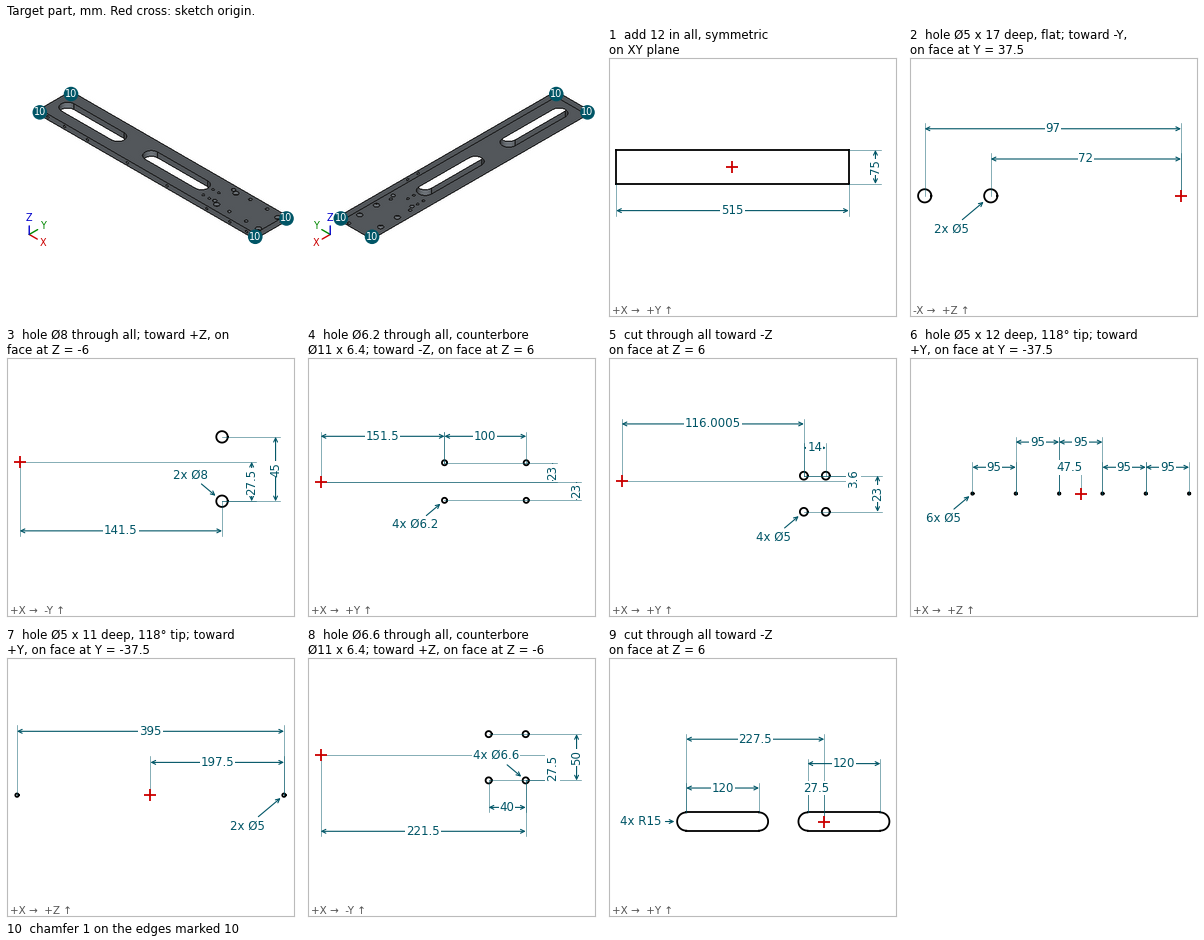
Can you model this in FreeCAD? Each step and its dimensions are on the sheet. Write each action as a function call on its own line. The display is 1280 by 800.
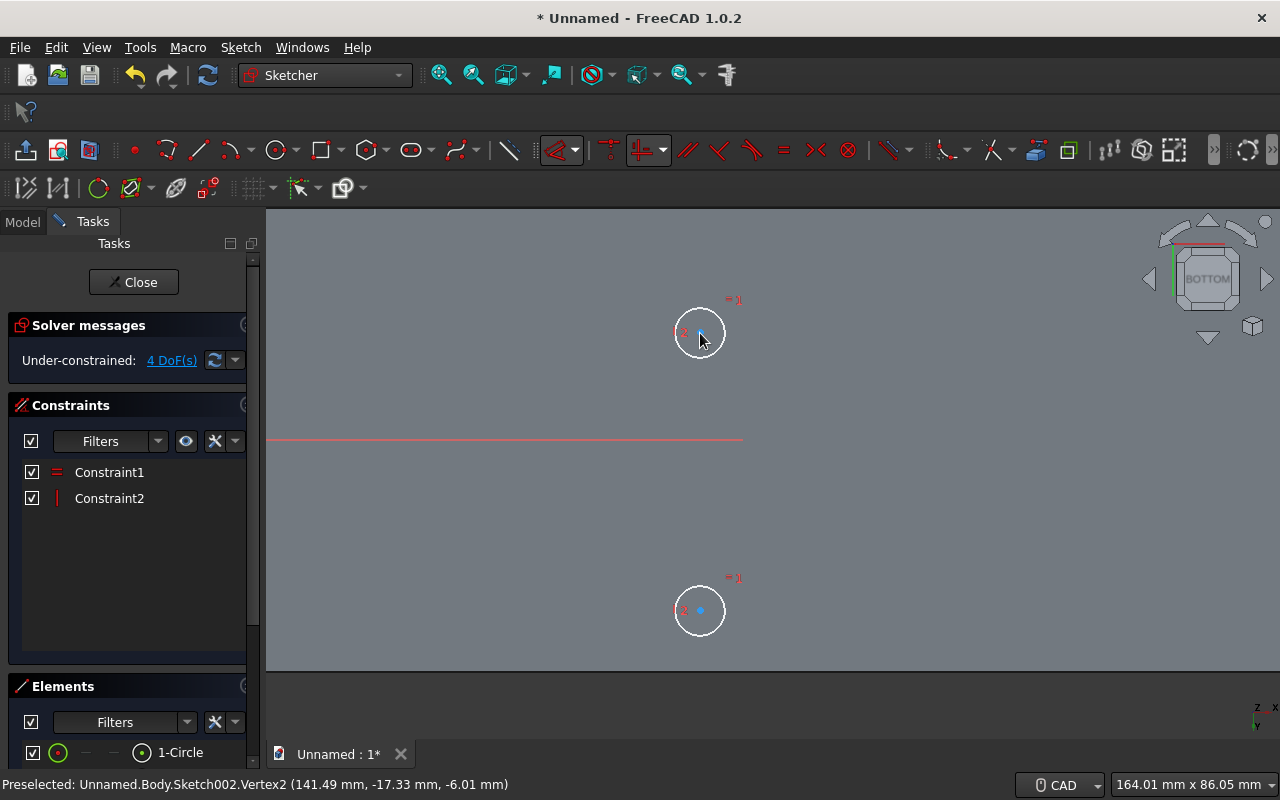
key(d)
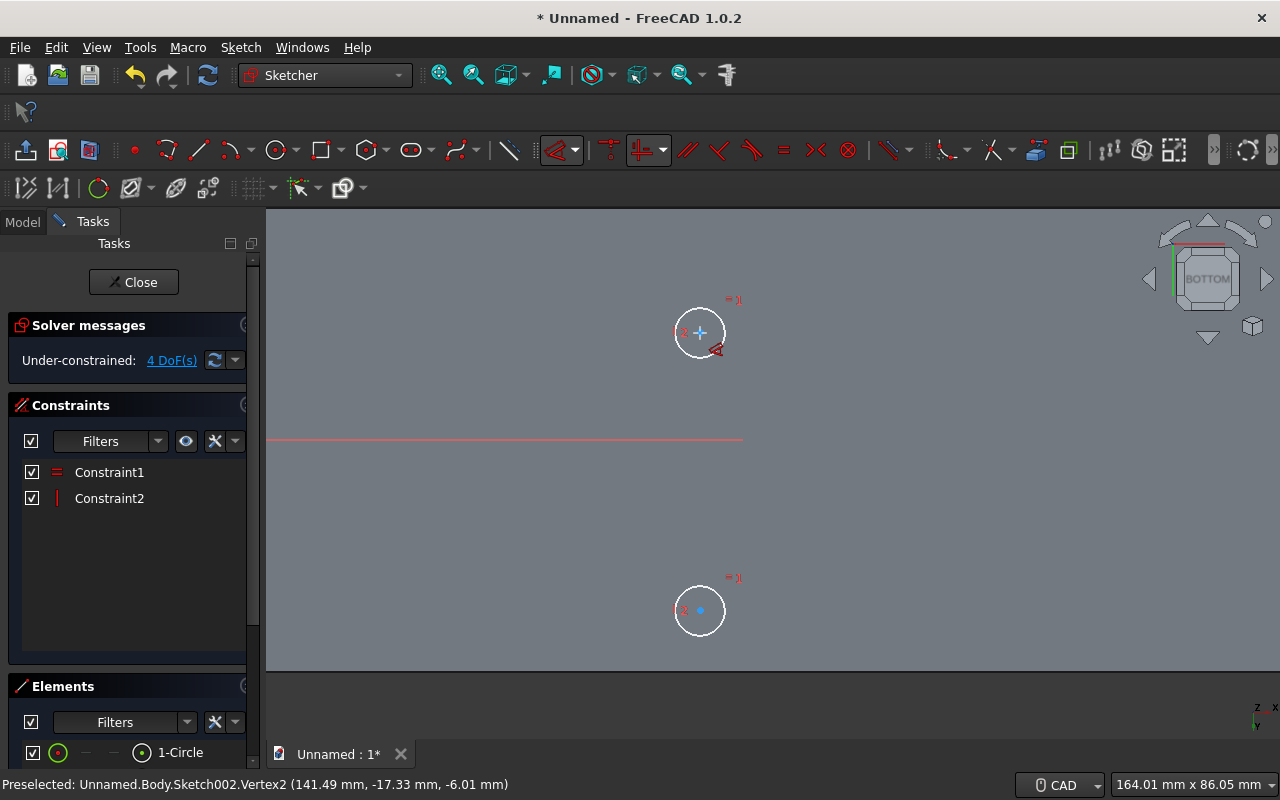
click(717, 593)
click(739, 570)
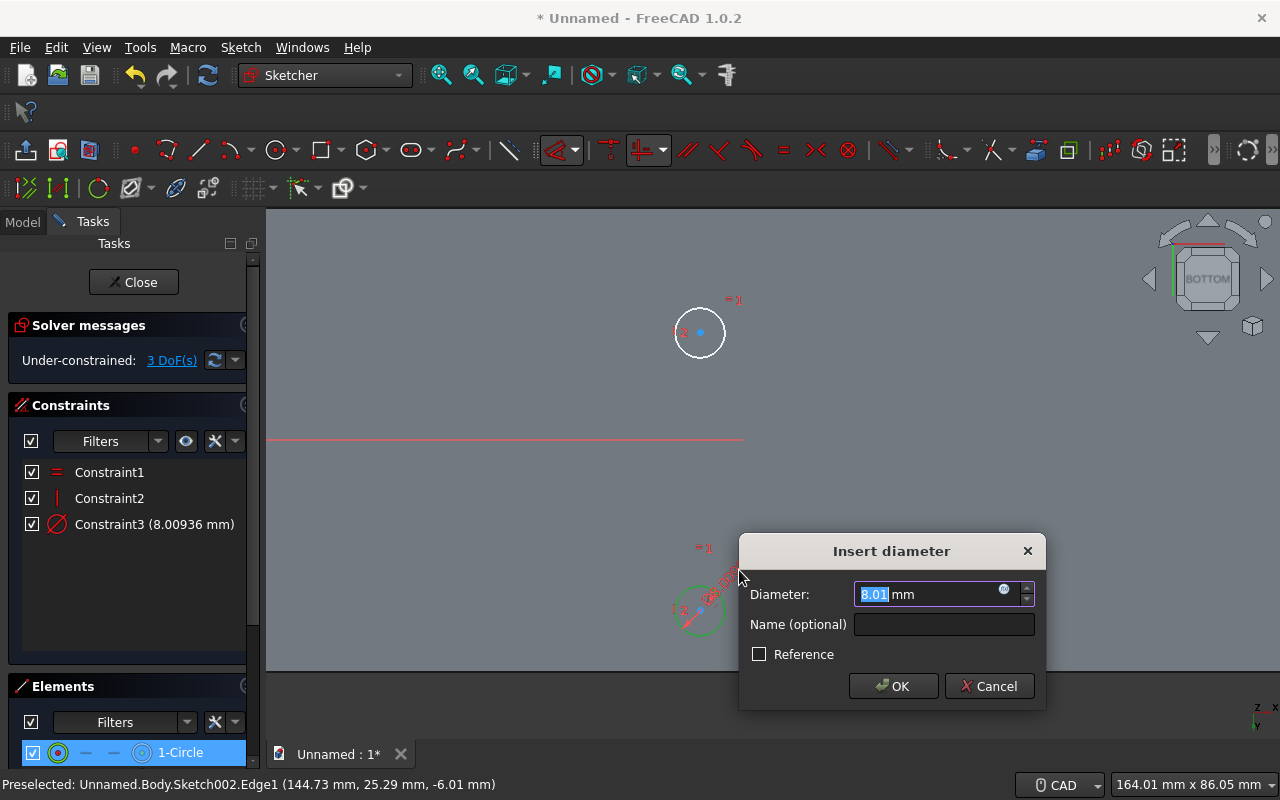
text(8)
key(Return)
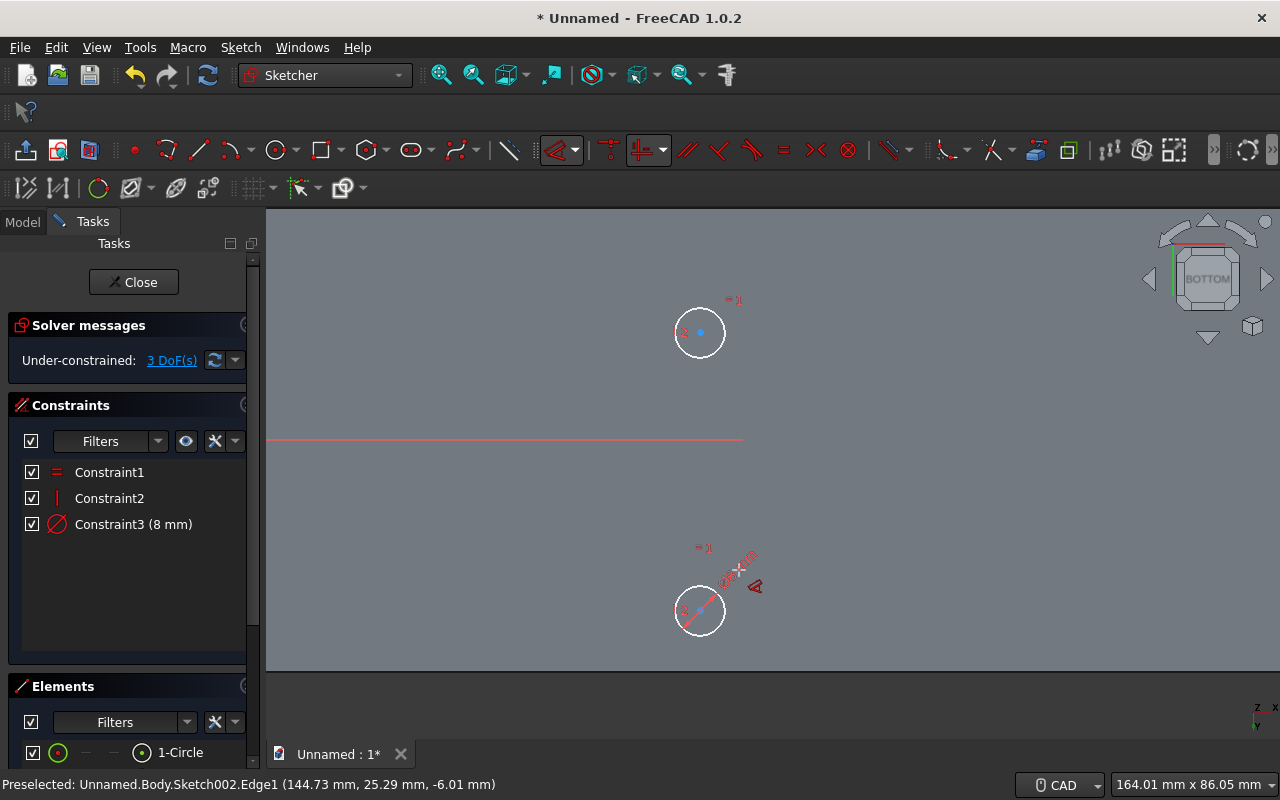
click(700, 611)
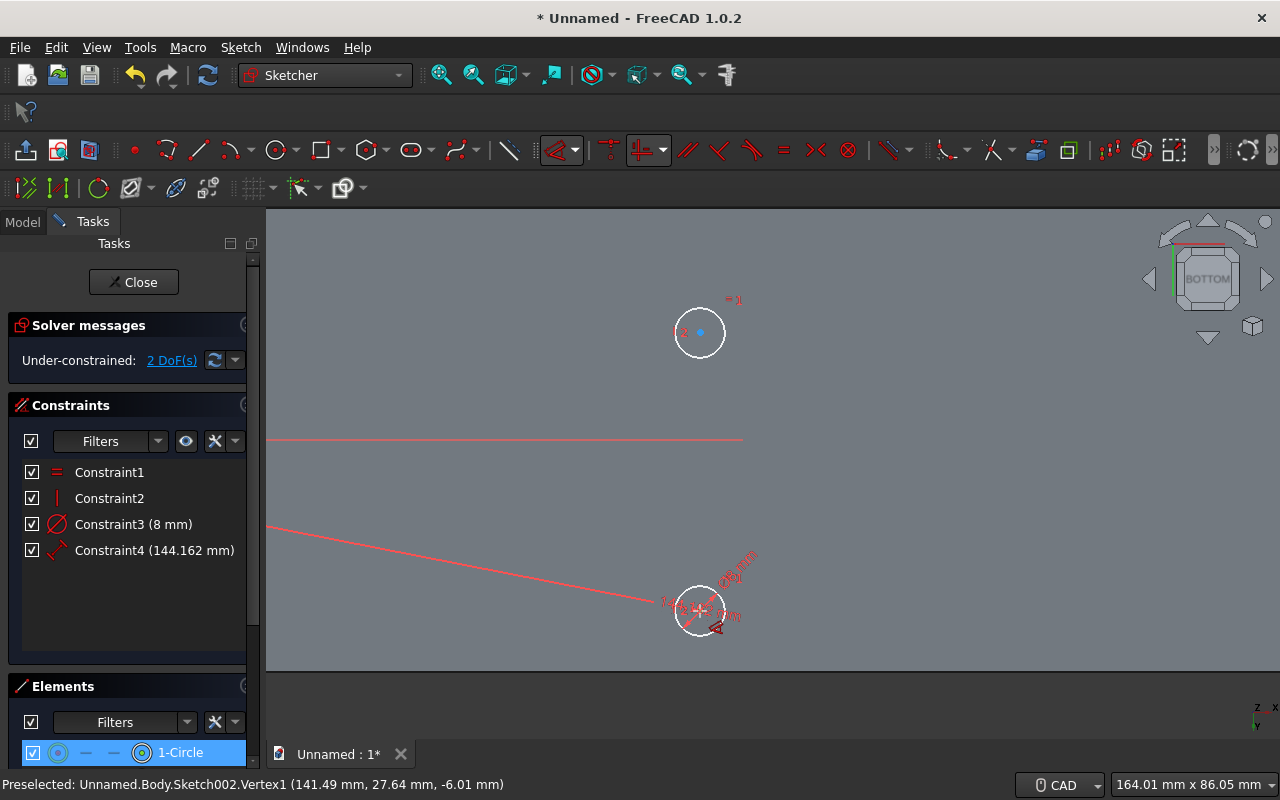
click(700, 333)
click(666, 472)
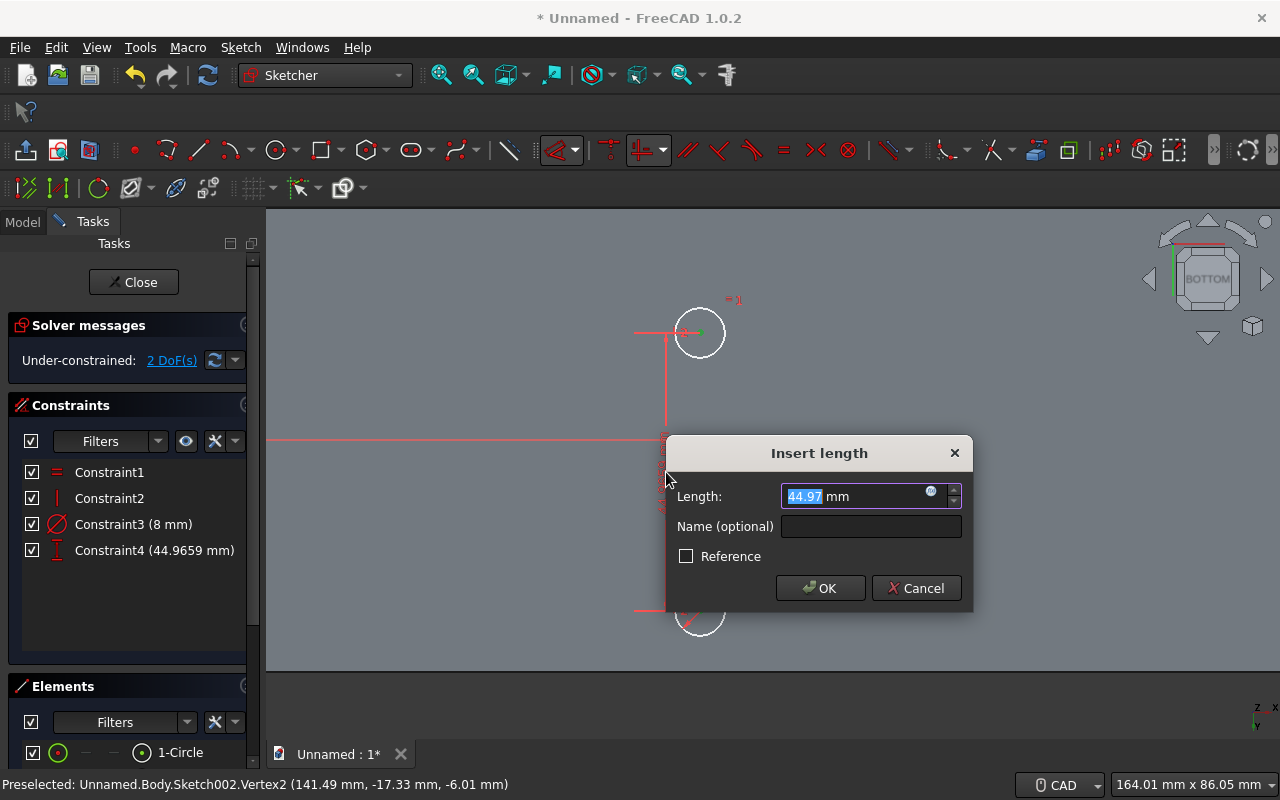
text(45)
key(Return)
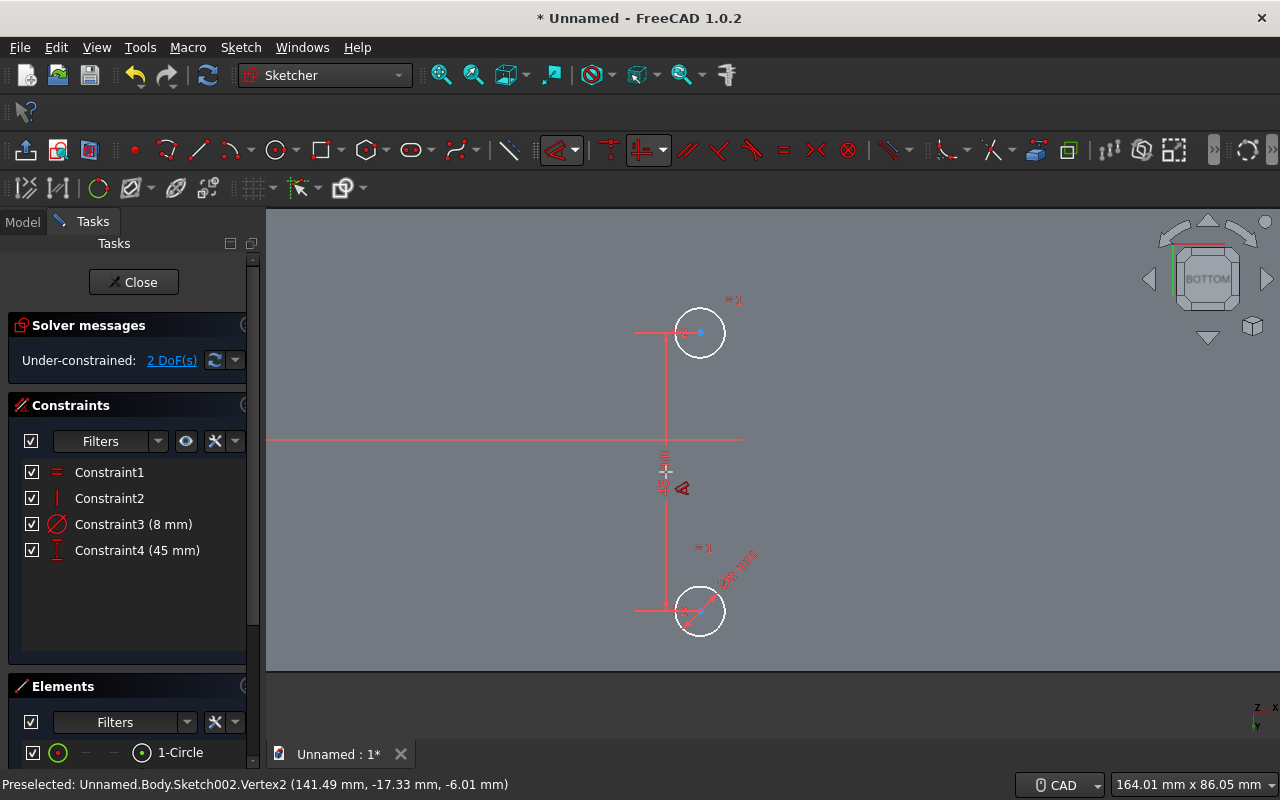
click(700, 611)
click(734, 526)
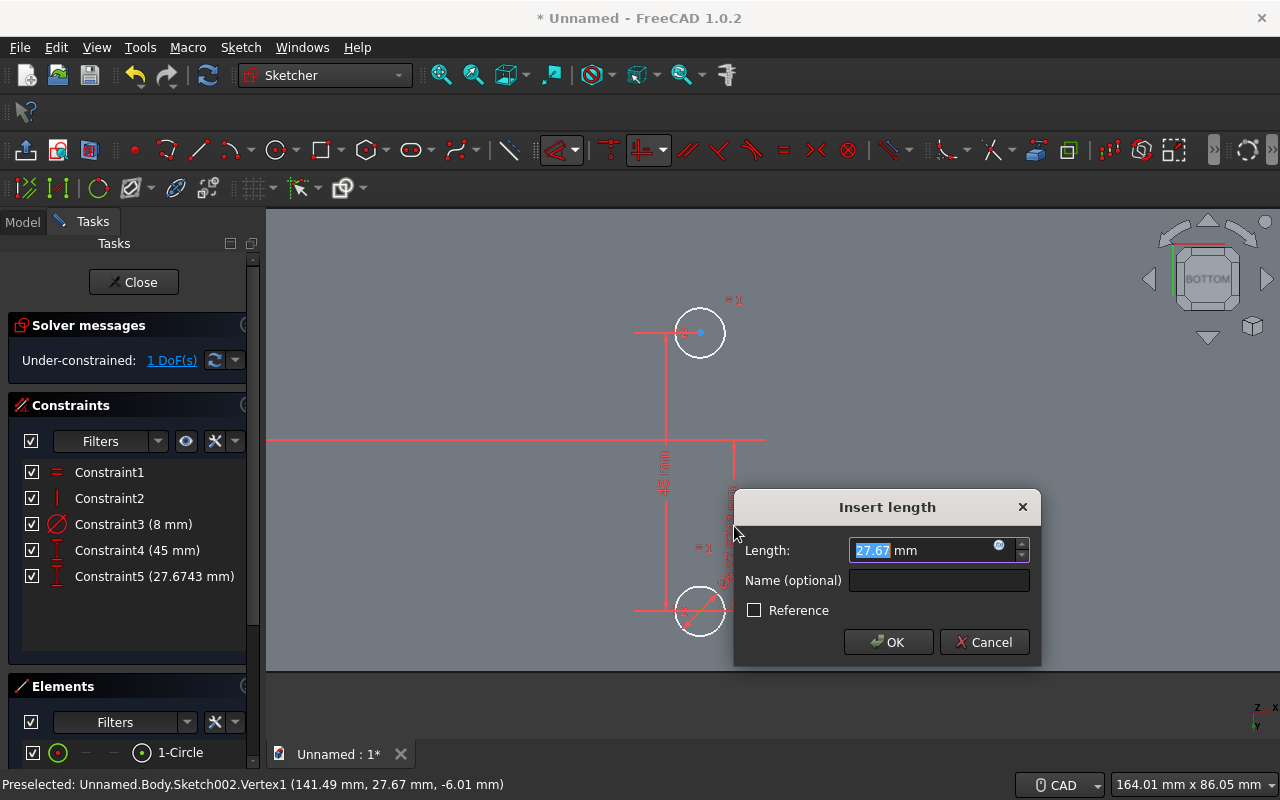
text(27.5)
key(Return)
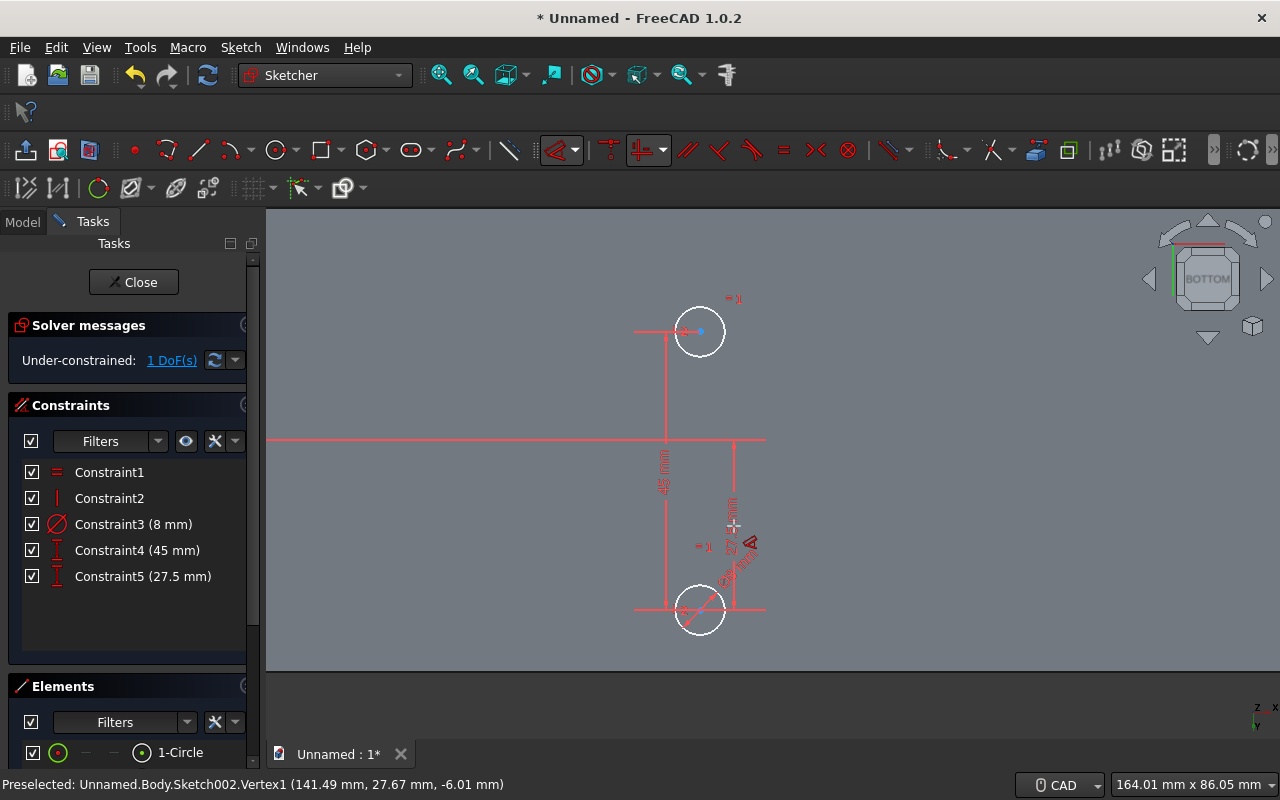
click(700, 610)
click(497, 644)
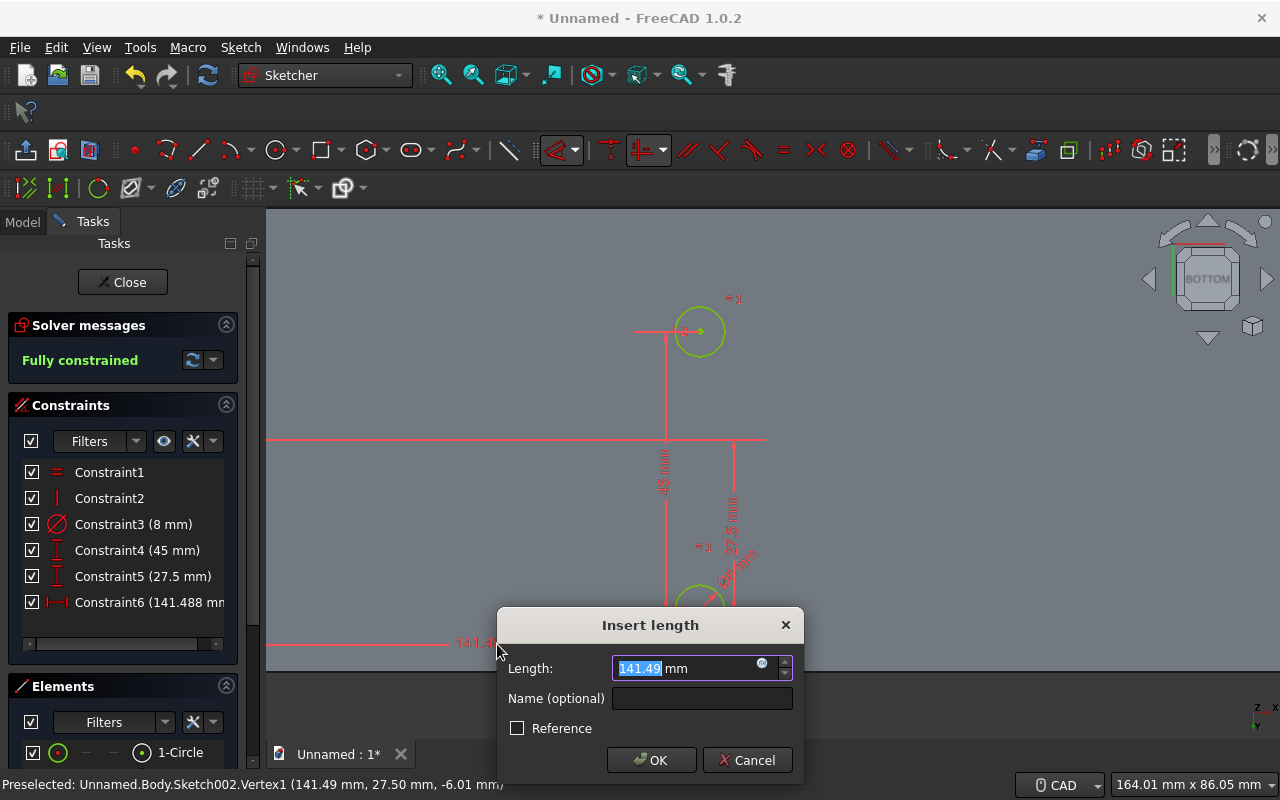
text(141.5)
key(Return)
key(Escape)